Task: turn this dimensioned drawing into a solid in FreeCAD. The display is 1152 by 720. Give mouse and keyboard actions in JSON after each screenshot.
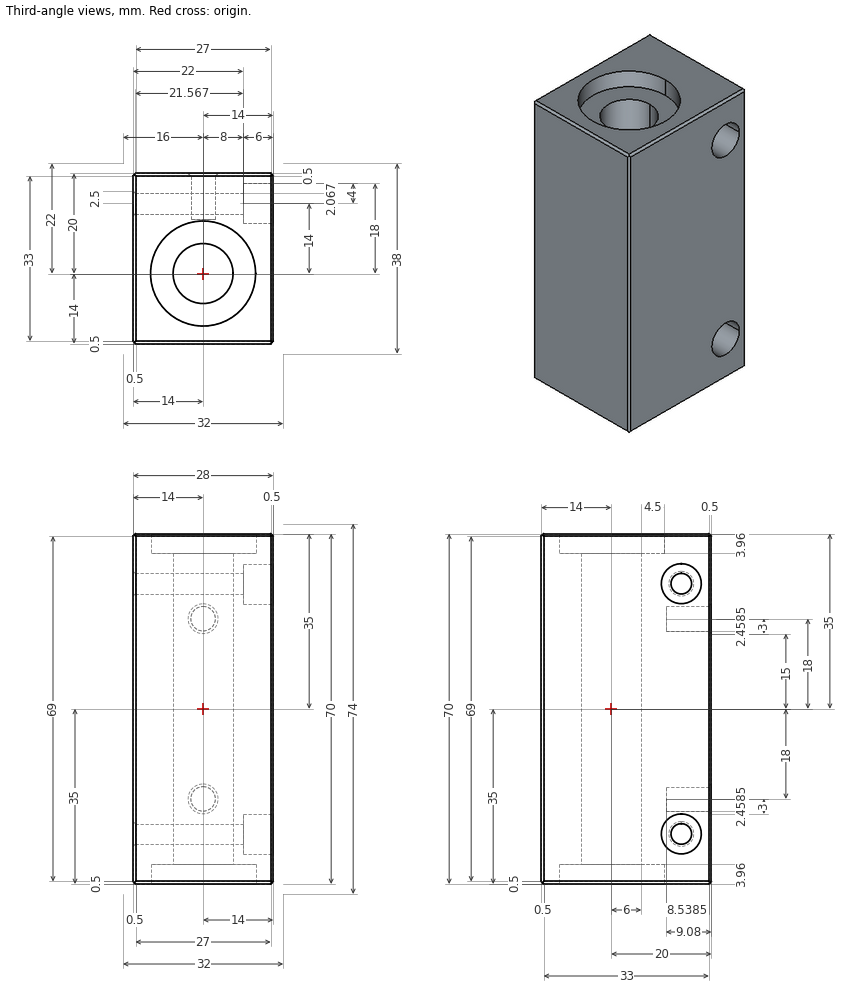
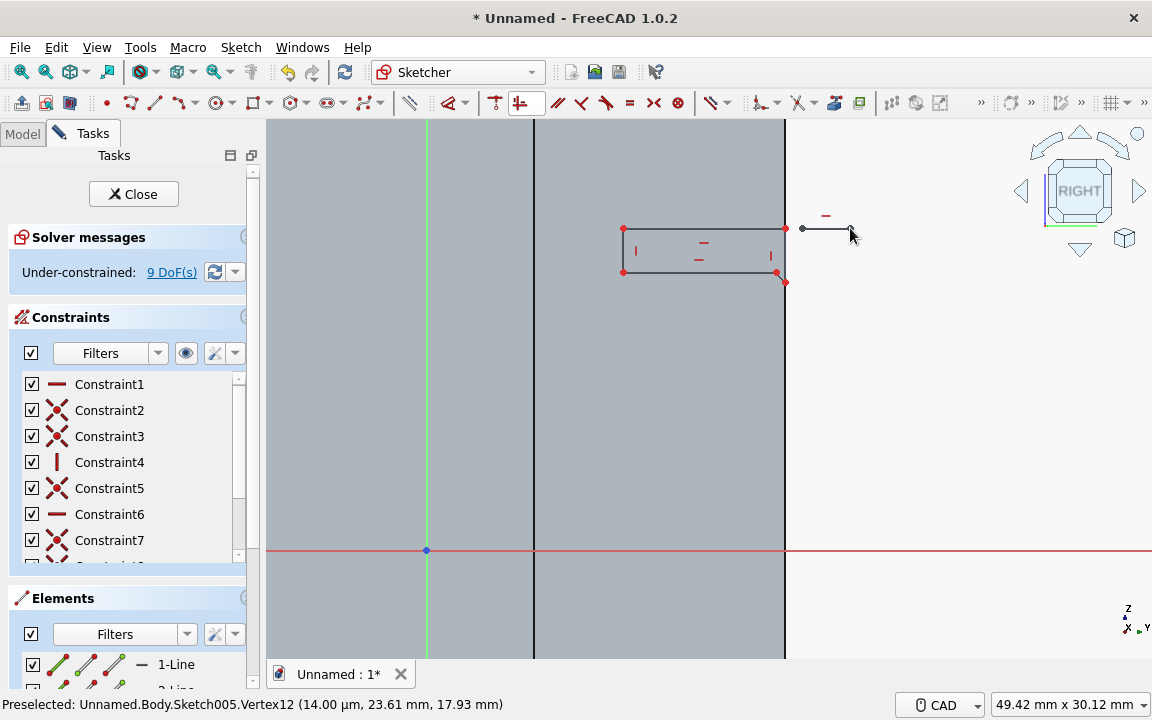
{"action": "left_click", "coordinate": [816, 229]}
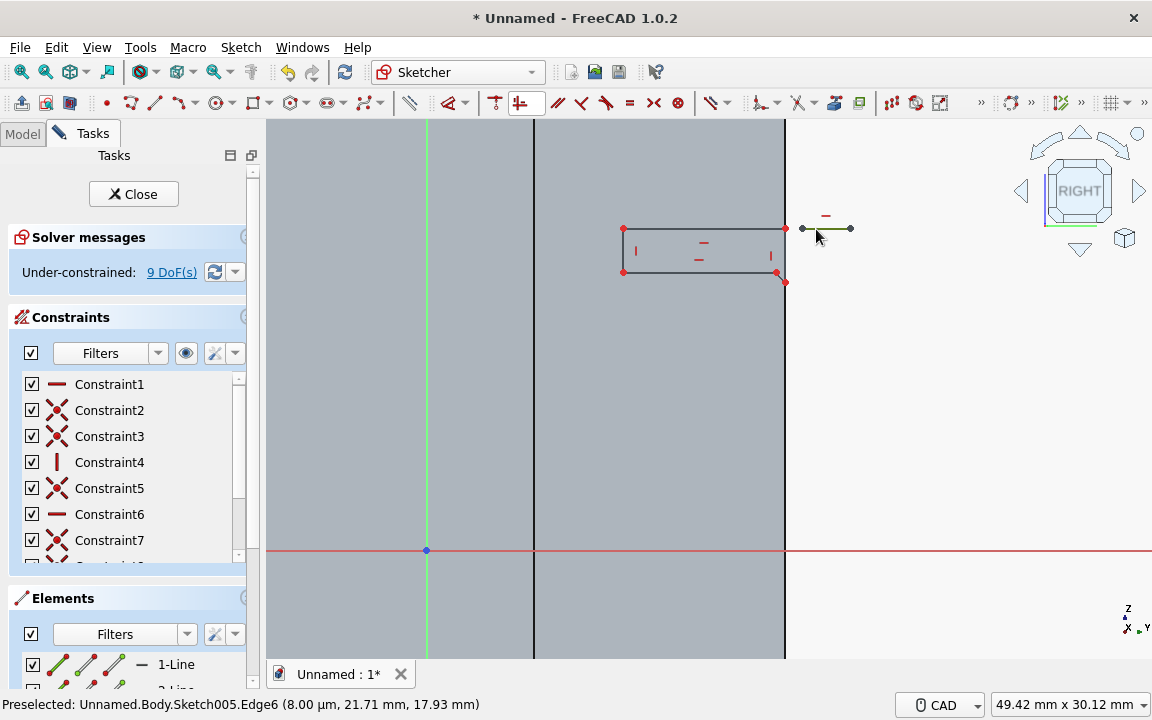
{"action": "left_click", "coordinate": [410, 104]}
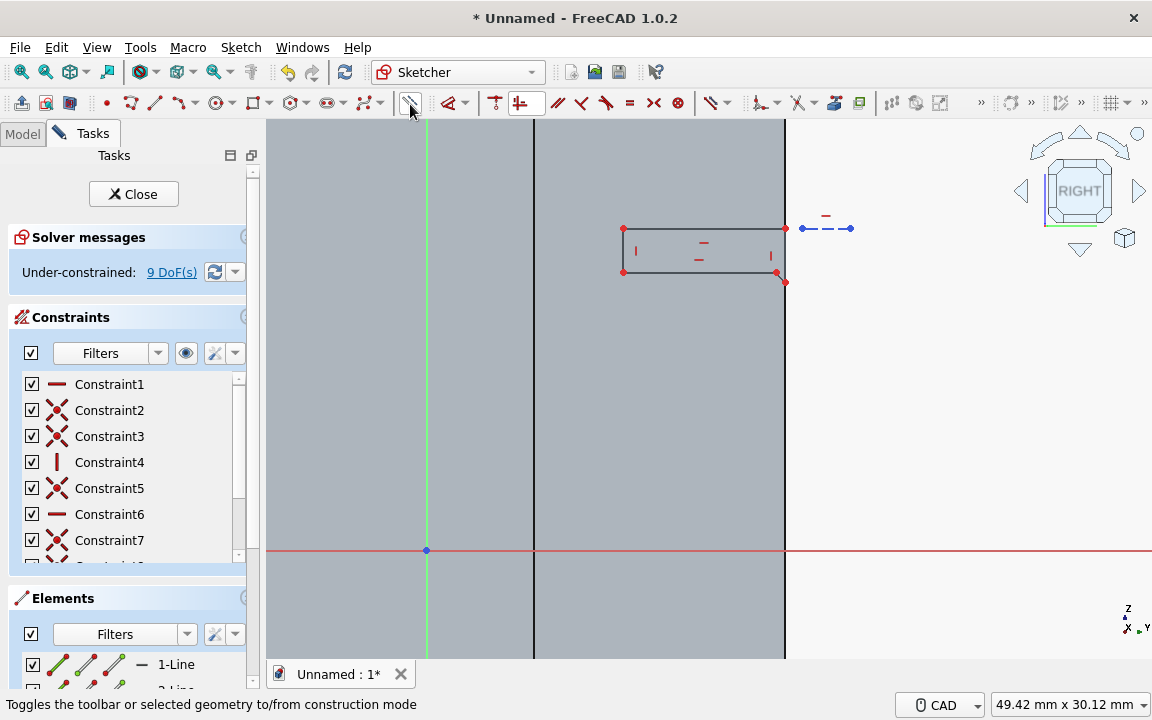
{"action": "left_click", "coordinate": [448, 104]}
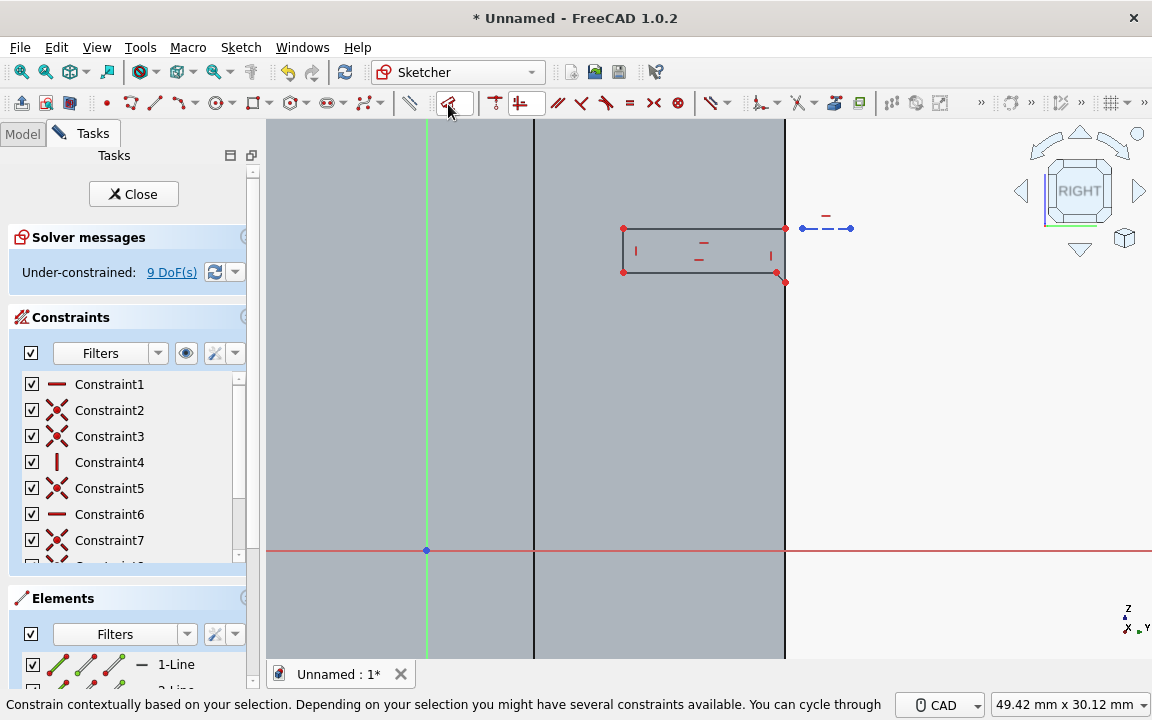
{"action": "scroll", "coordinate": [785, 267], "scroll_direction": "up", "scroll_amount": 2}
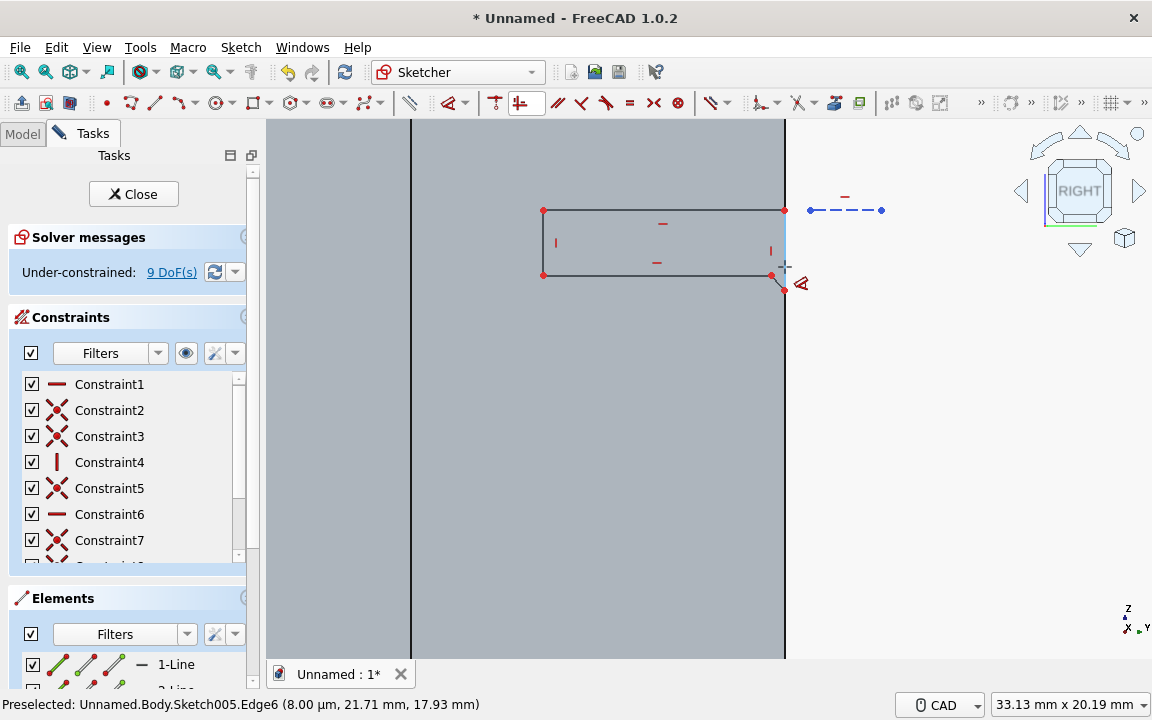
{"action": "left_click", "coordinate": [785, 267]}
{"action": "left_click", "coordinate": [819, 250]}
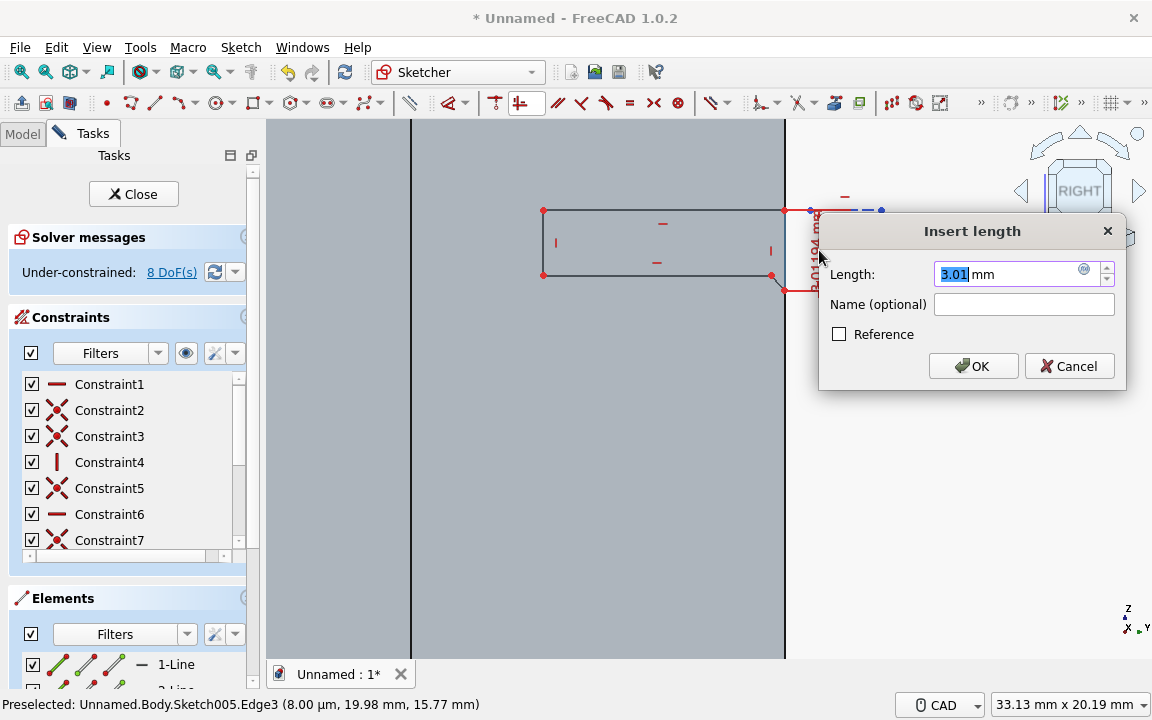
{"action": "type", "text": "3"}
{"action": "key", "text": "Return"}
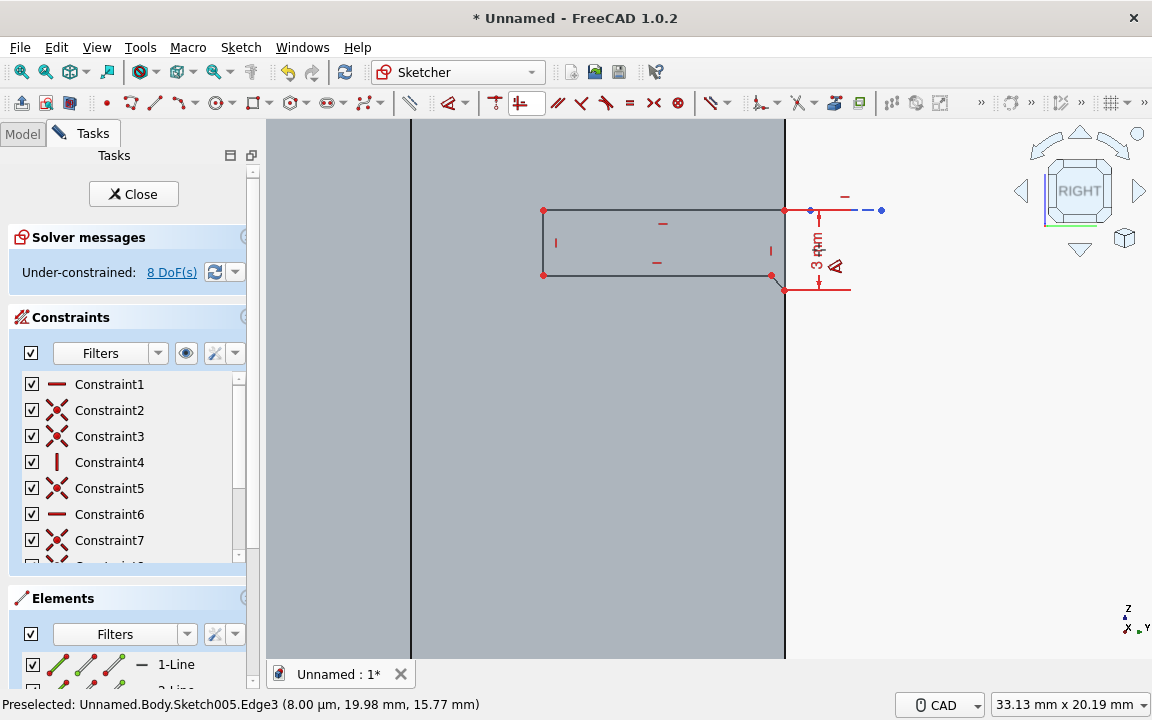
{"action": "left_click", "coordinate": [785, 290]}
{"action": "left_click", "coordinate": [426, 256]}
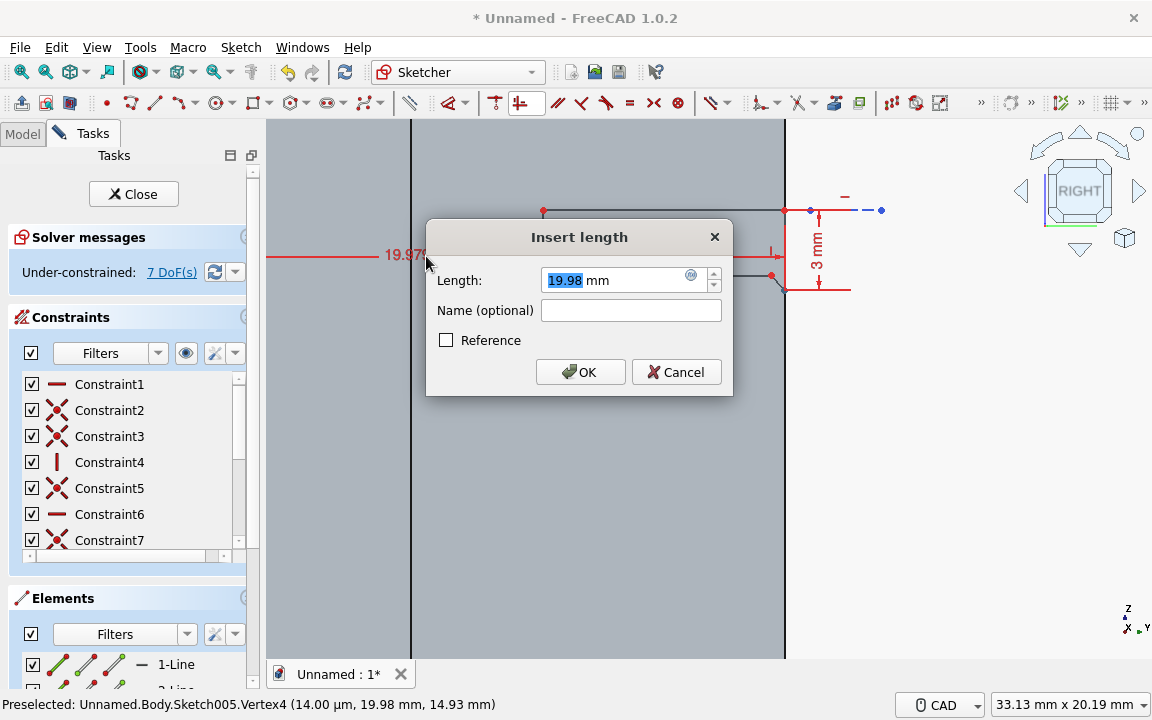
{"action": "type", "text": "20"}
{"action": "key", "text": "Return"}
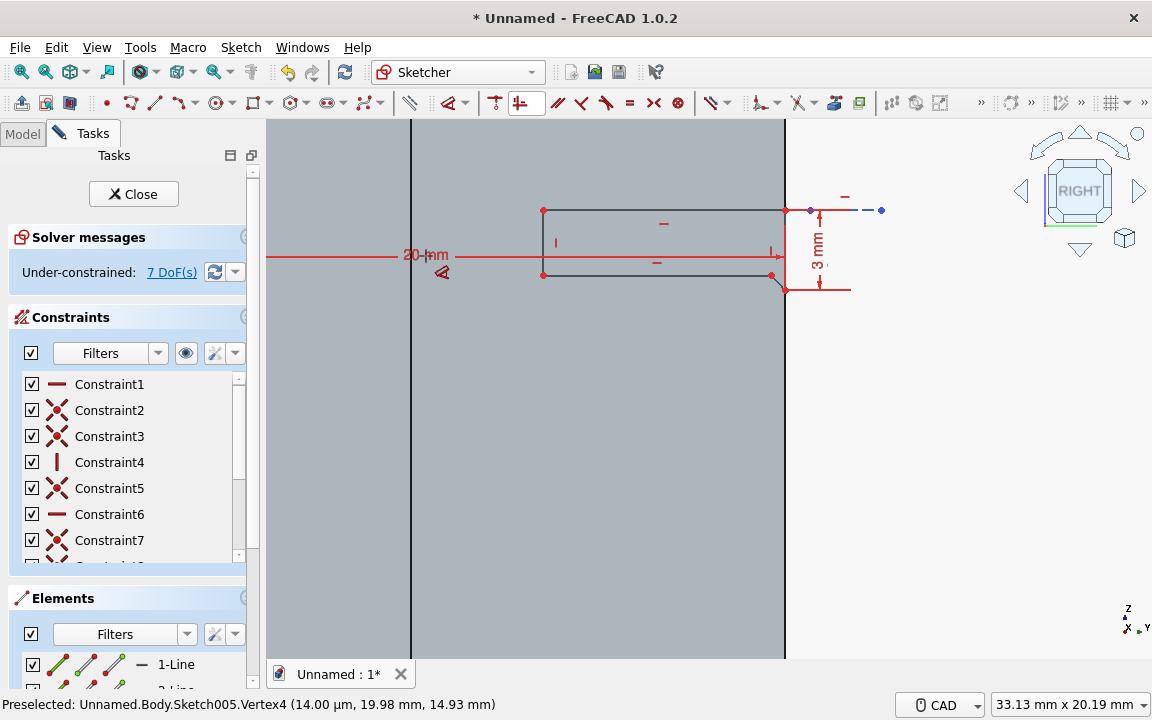
{"action": "left_click", "coordinate": [785, 290]}
{"action": "left_click", "coordinate": [819, 461]}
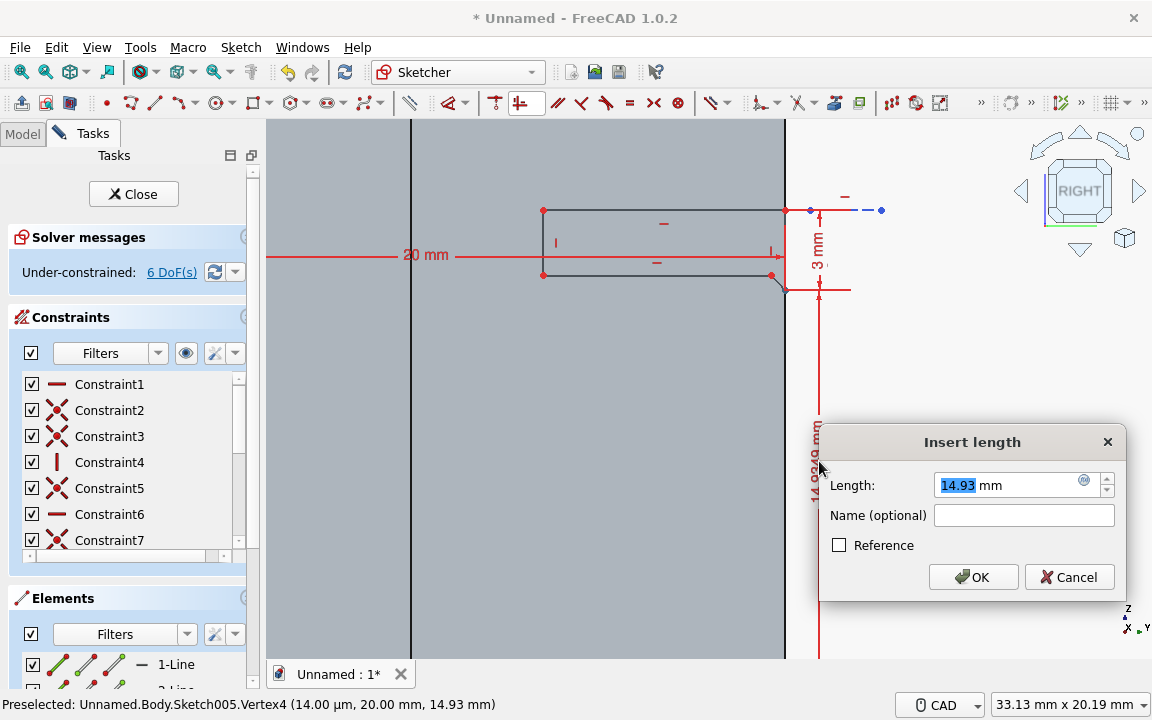
{"action": "type", "text": "15"}
{"action": "key", "text": "Return"}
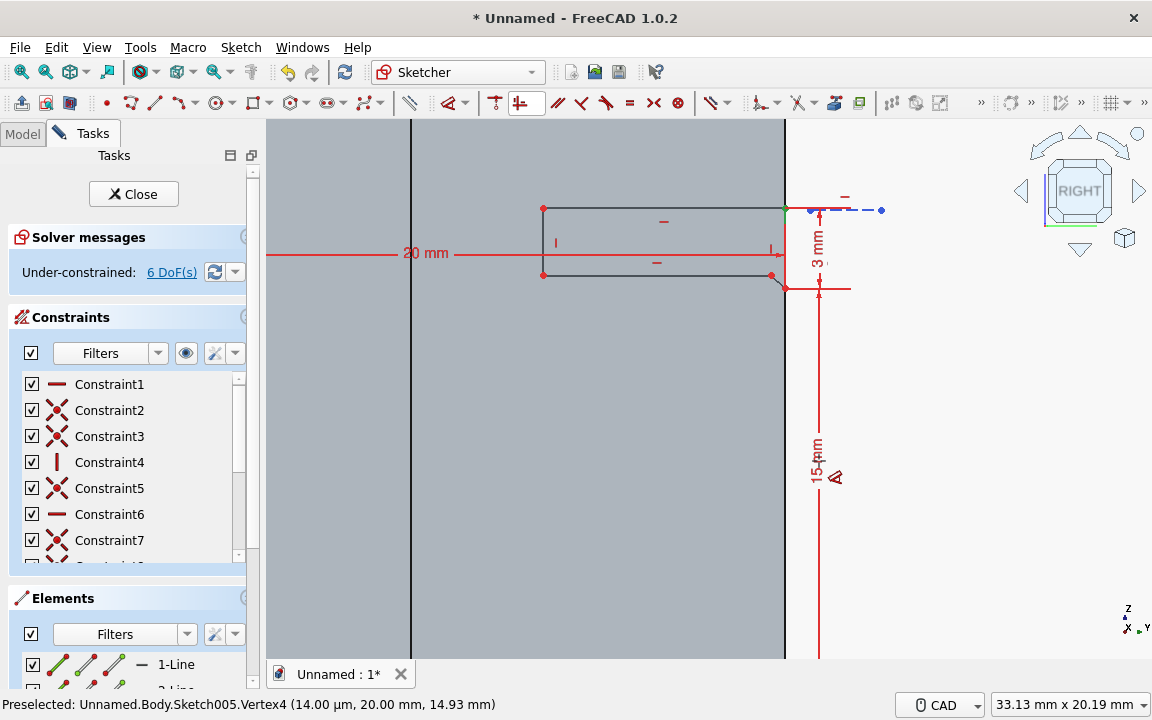
{"action": "left_click", "coordinate": [810, 210]}
{"action": "left_click", "coordinate": [844, 421]}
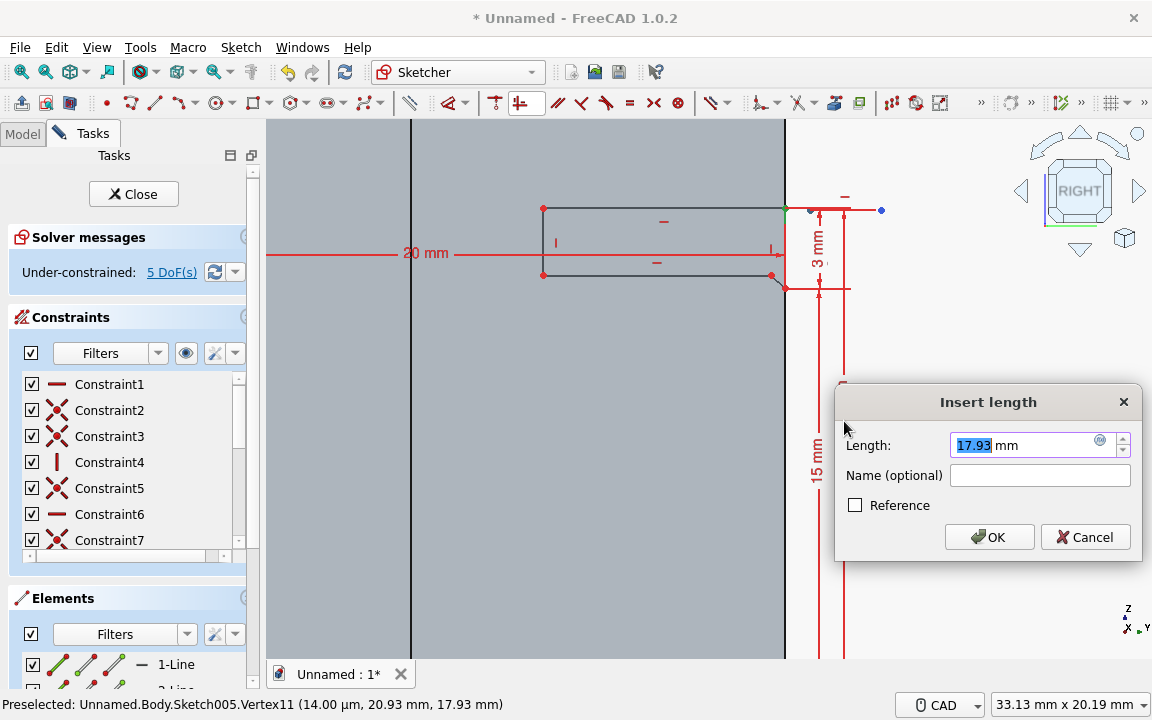
{"action": "type", "text": "18"}
{"action": "key", "text": "Return"}